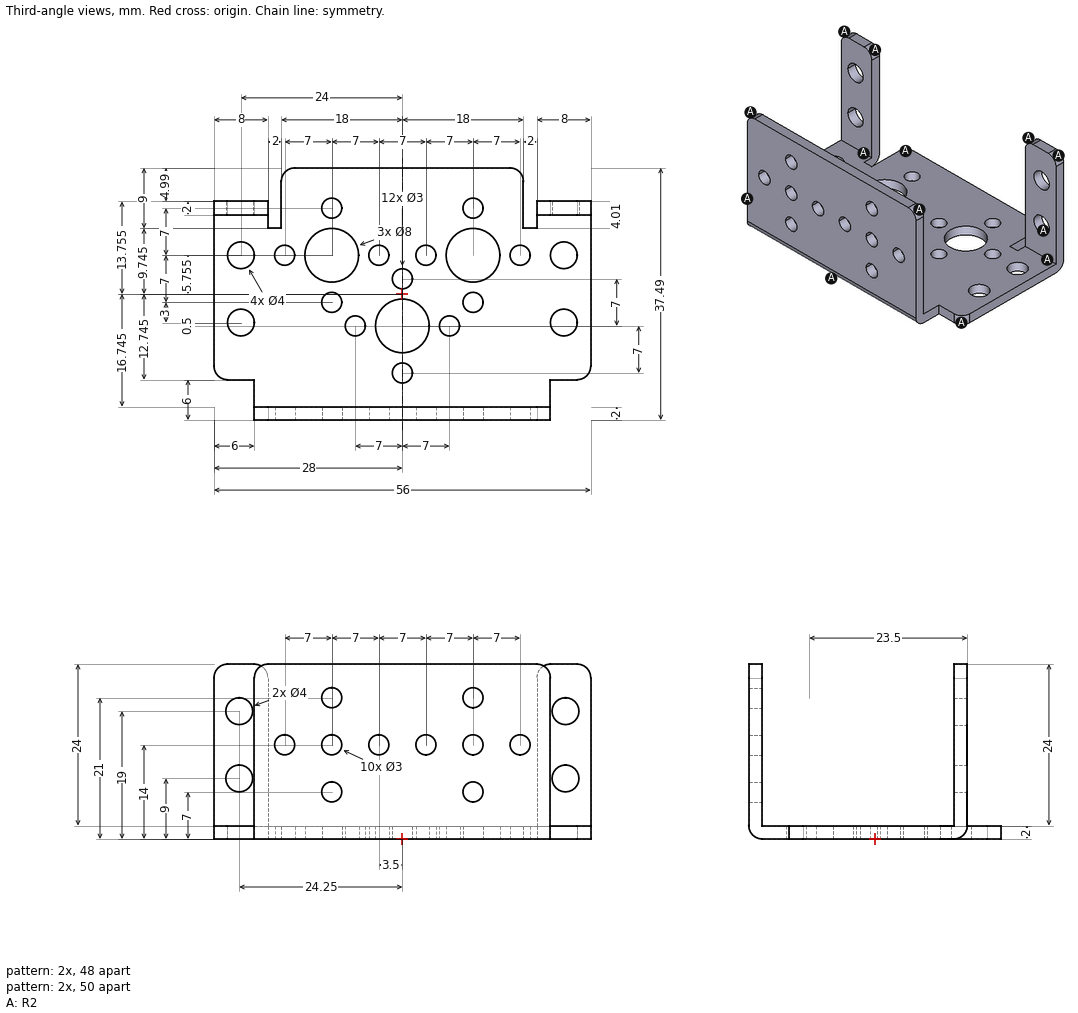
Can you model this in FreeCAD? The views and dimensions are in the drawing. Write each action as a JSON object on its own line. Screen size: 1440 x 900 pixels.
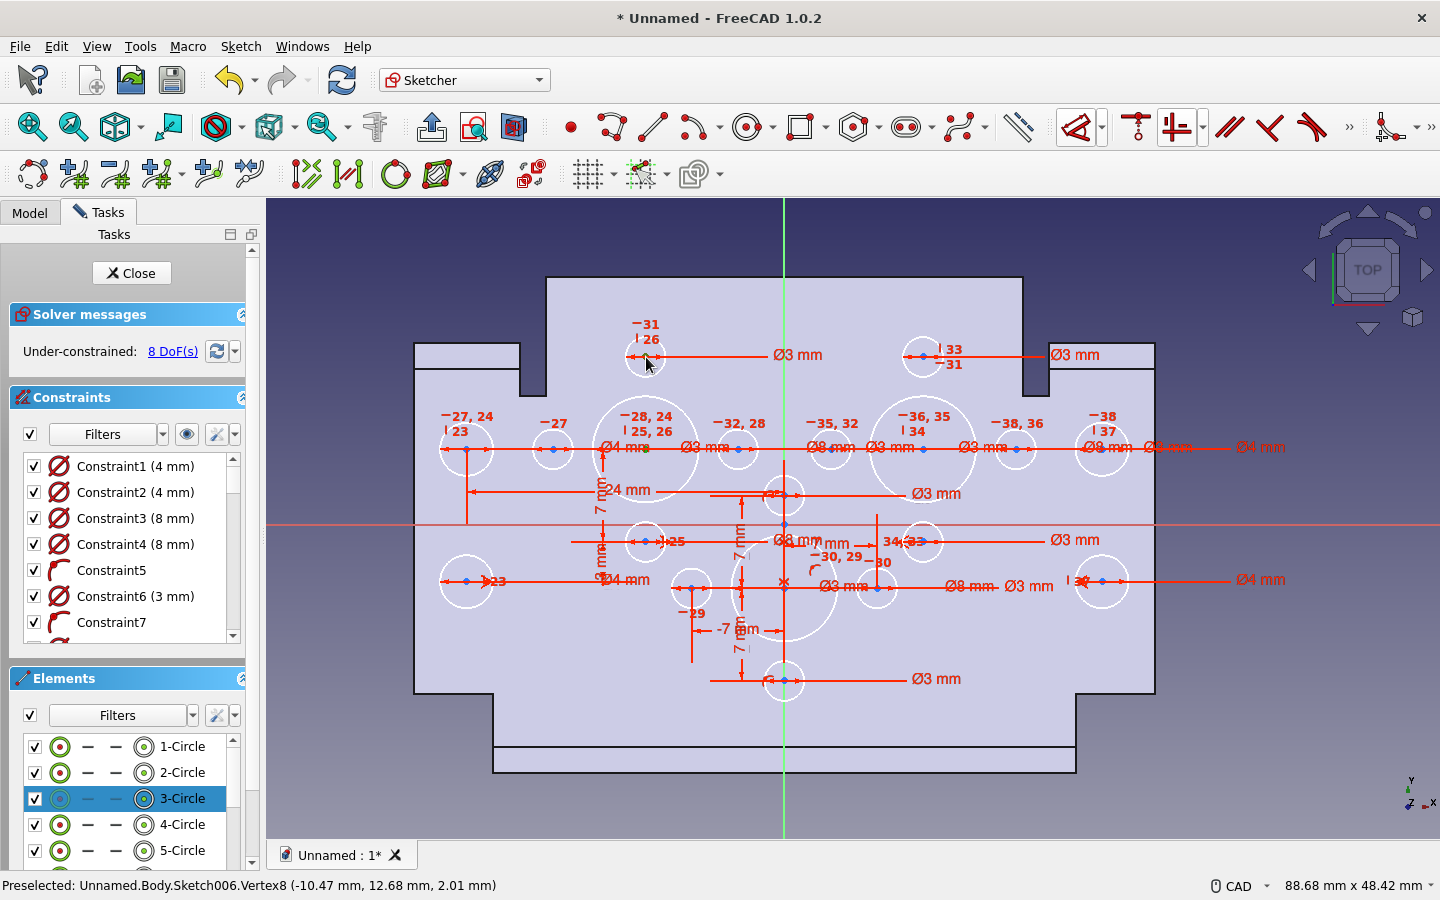
{"action": "key", "text": "i"}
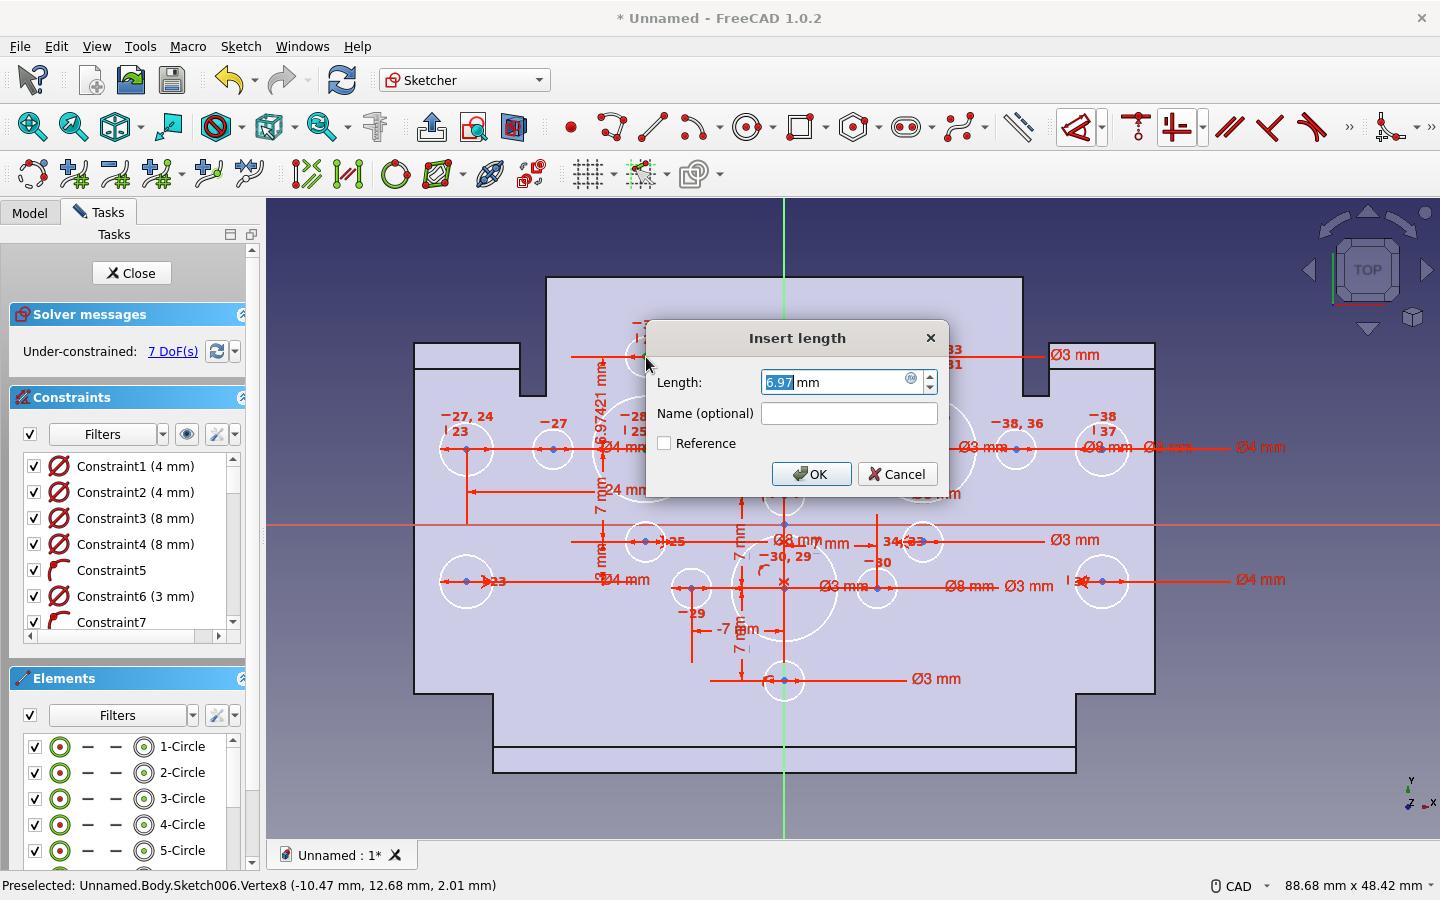
{"action": "type", "text": "7"}
{"action": "key", "text": "Return"}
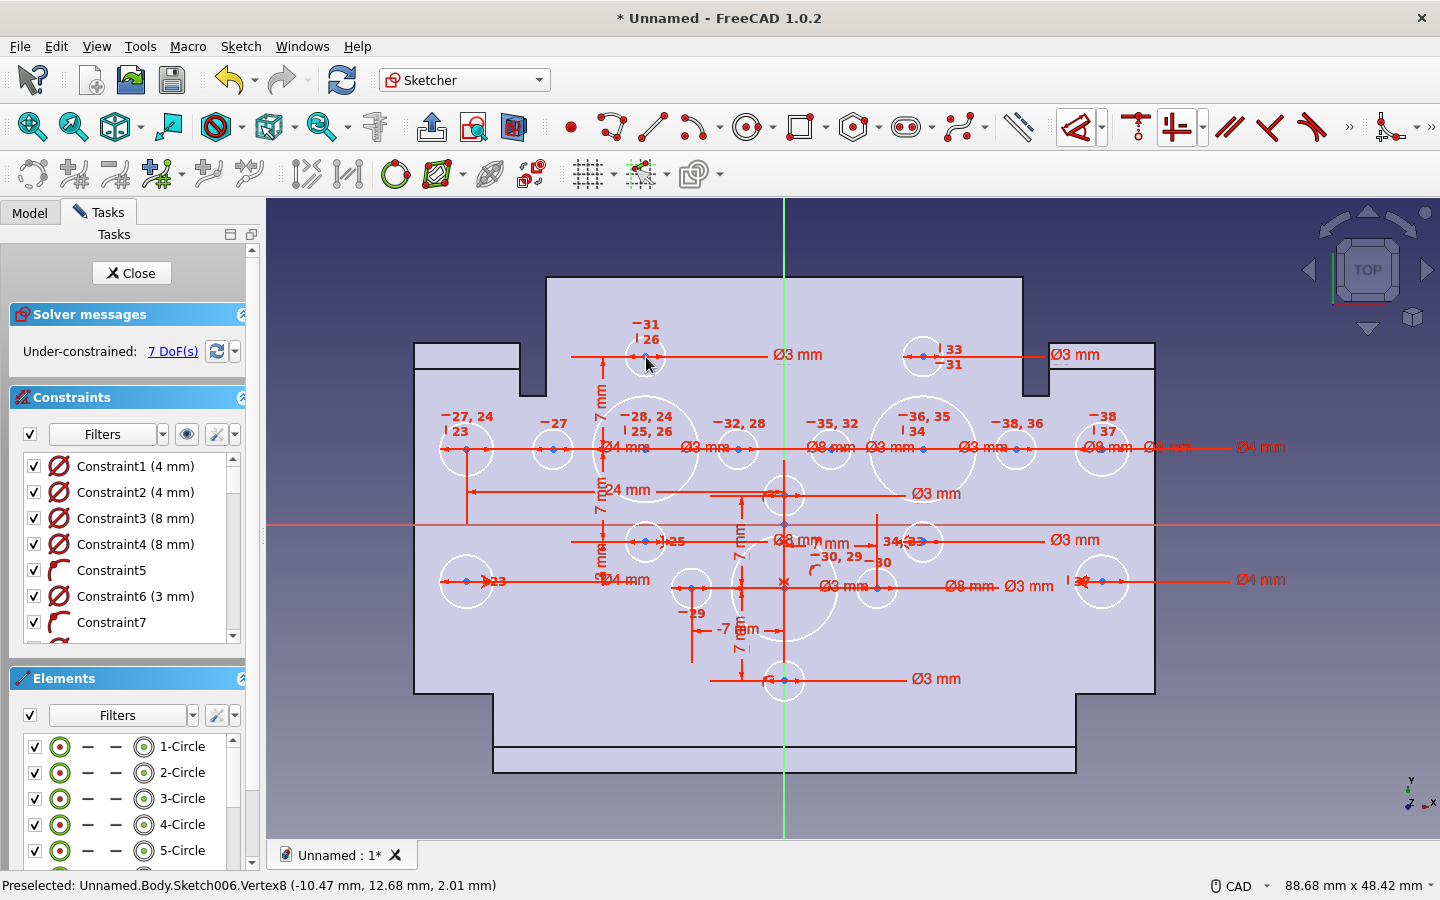
{"action": "left_click", "coordinate": [646, 449]}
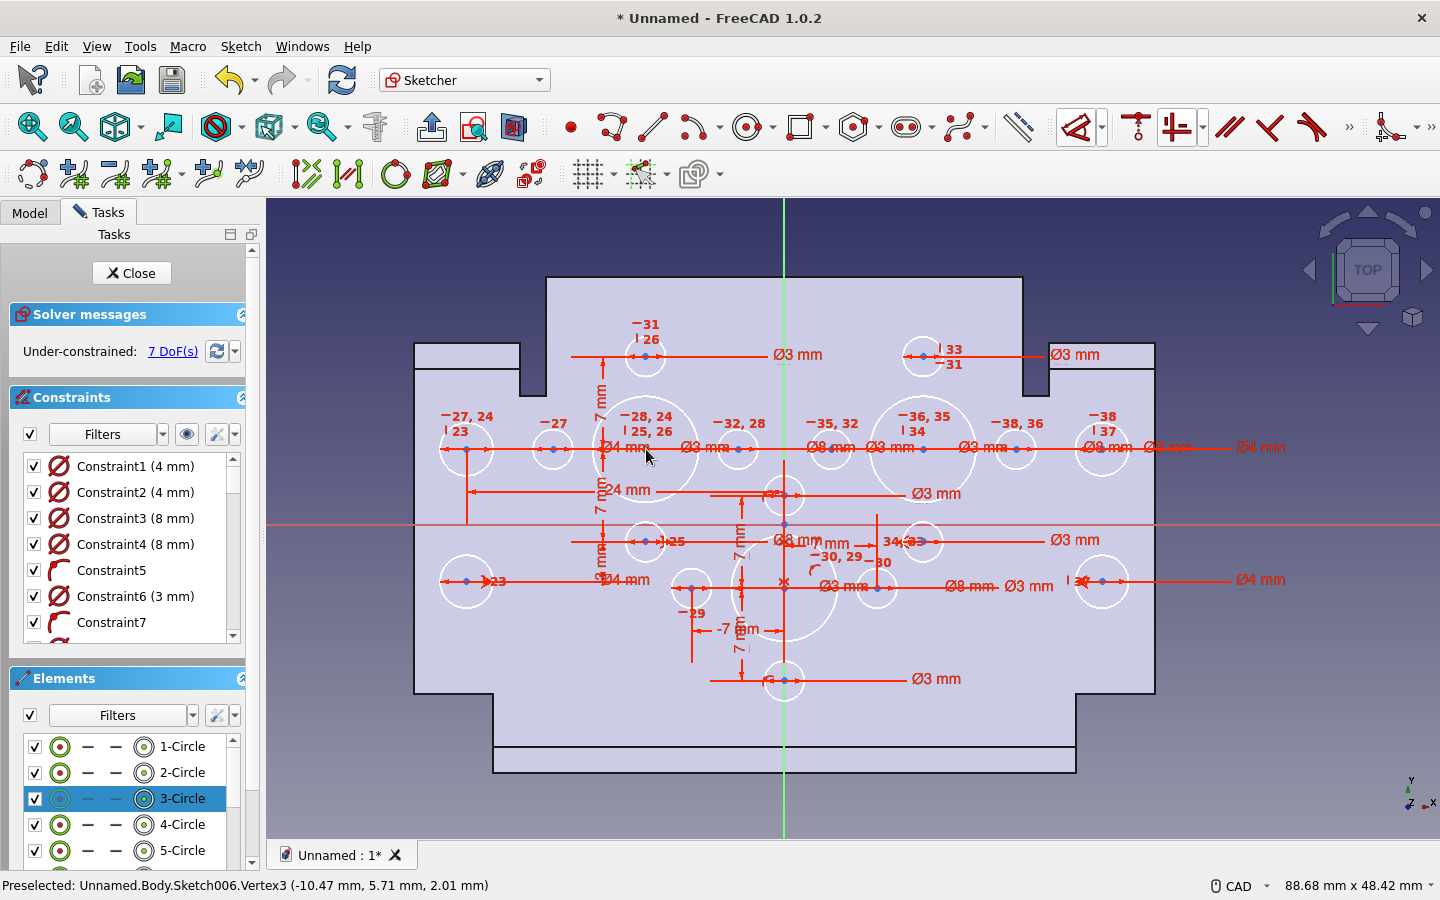
{"action": "left_click", "coordinate": [553, 449]}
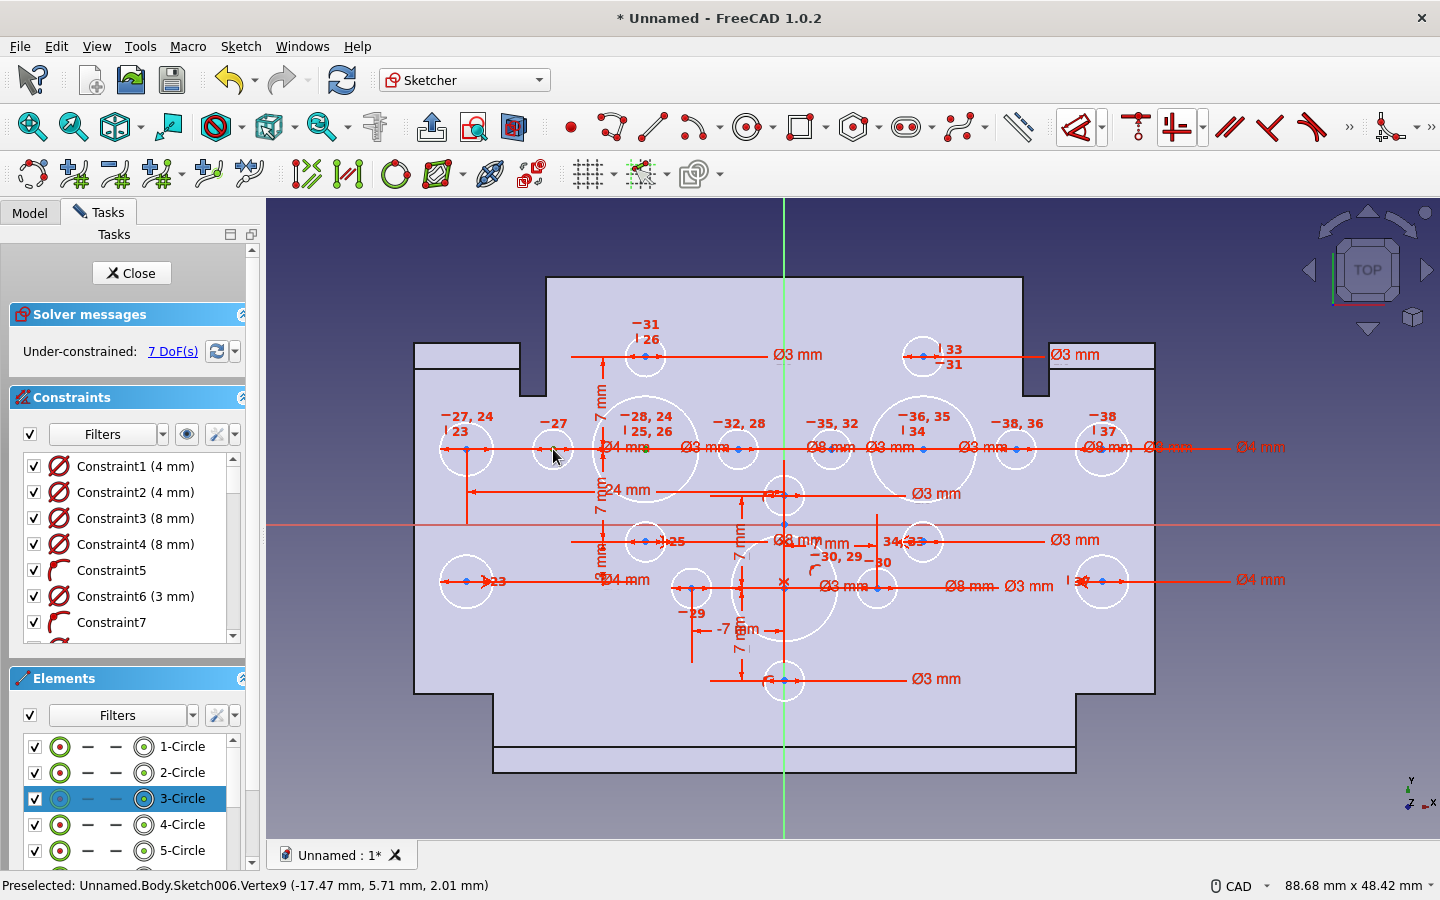
{"action": "key", "text": "l"}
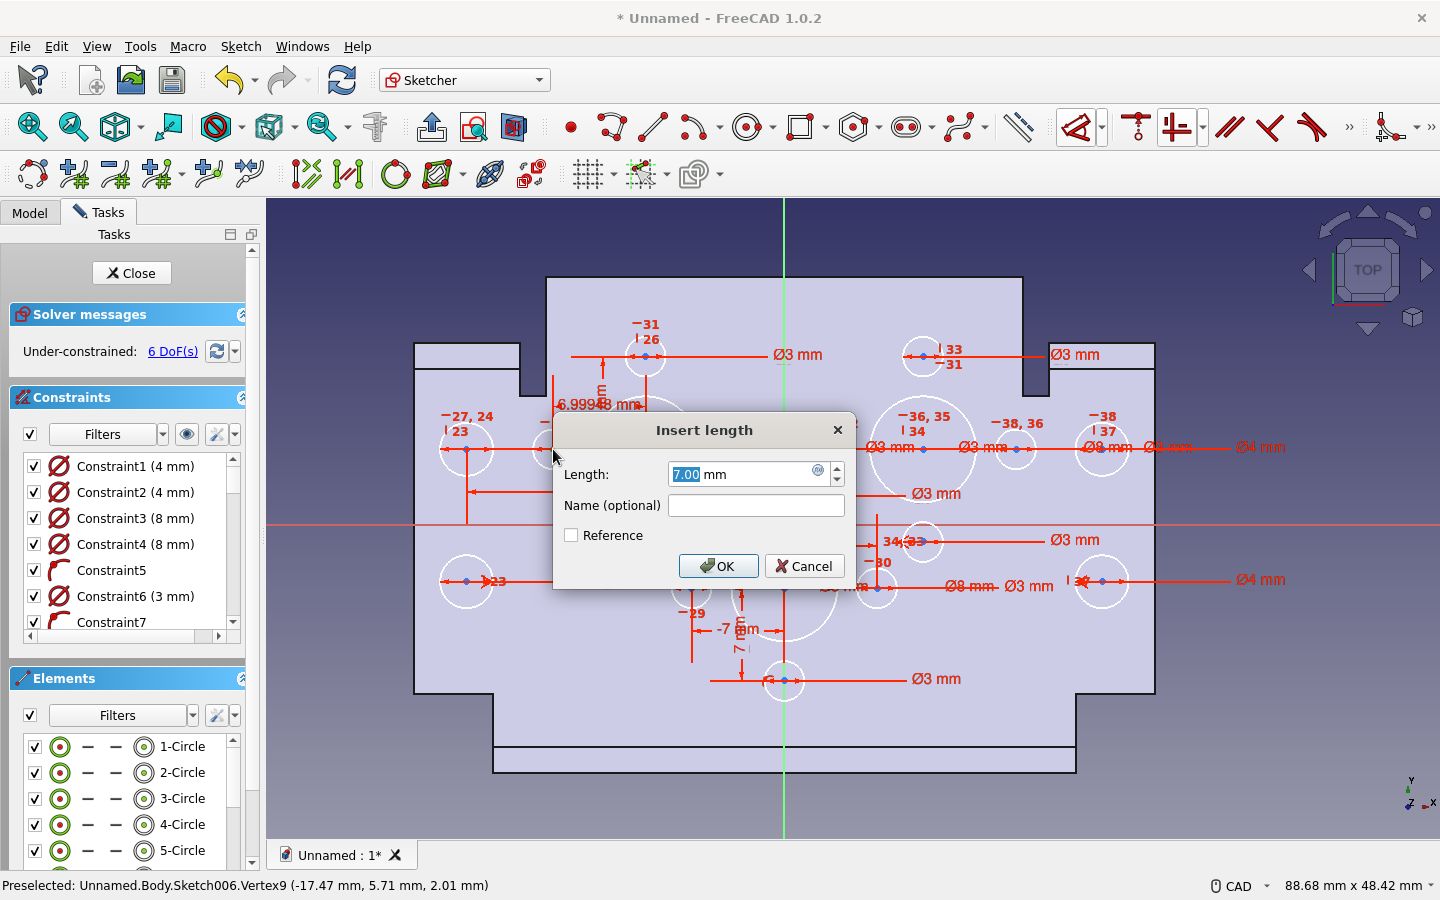
{"action": "type", "text": "7"}
{"action": "key", "text": "Return"}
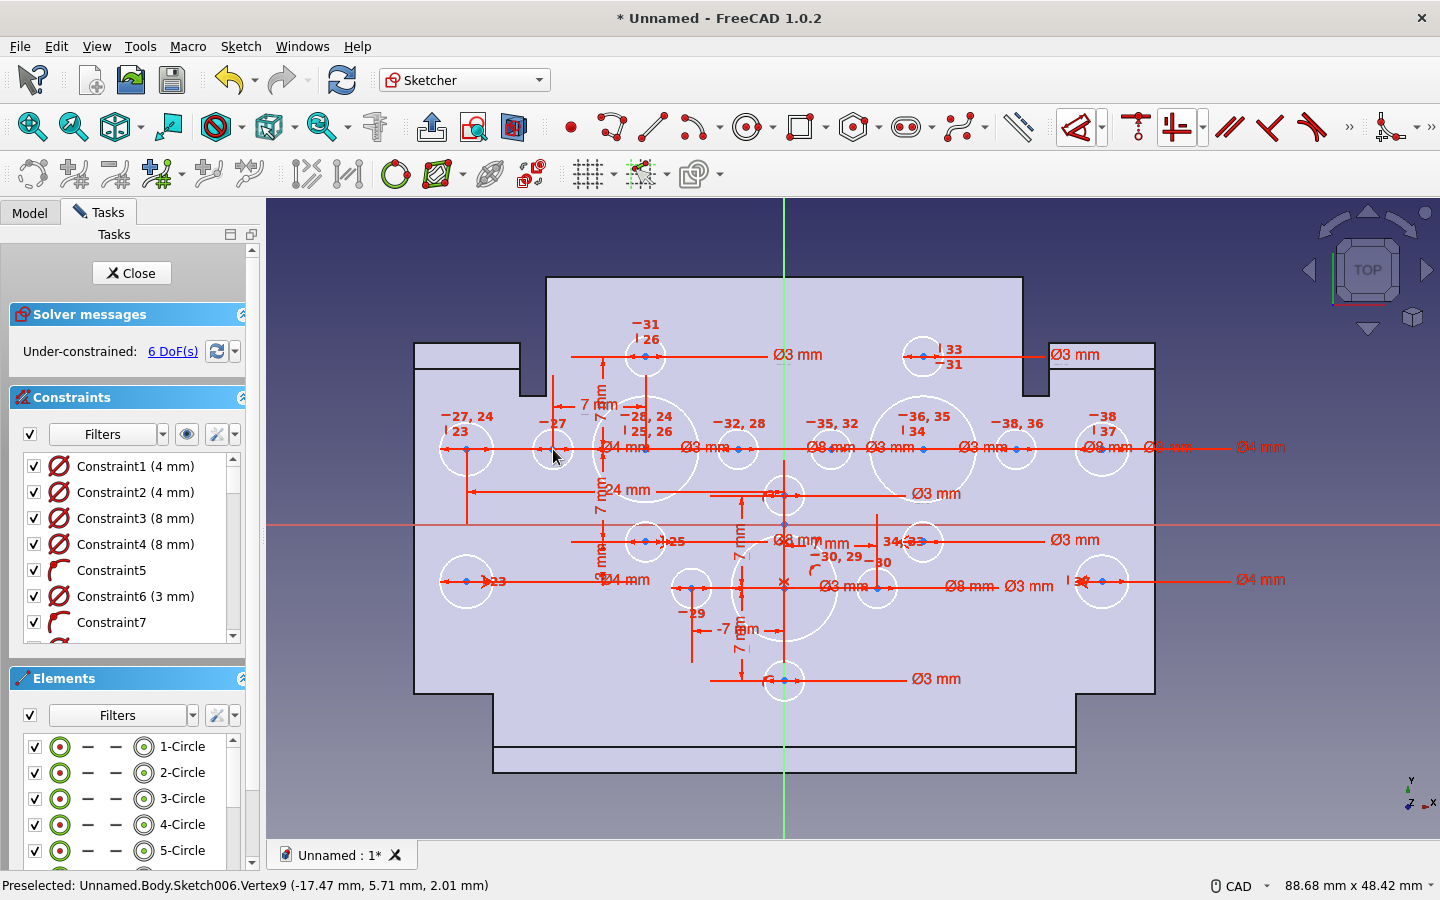
{"action": "left_click", "coordinate": [646, 449]}